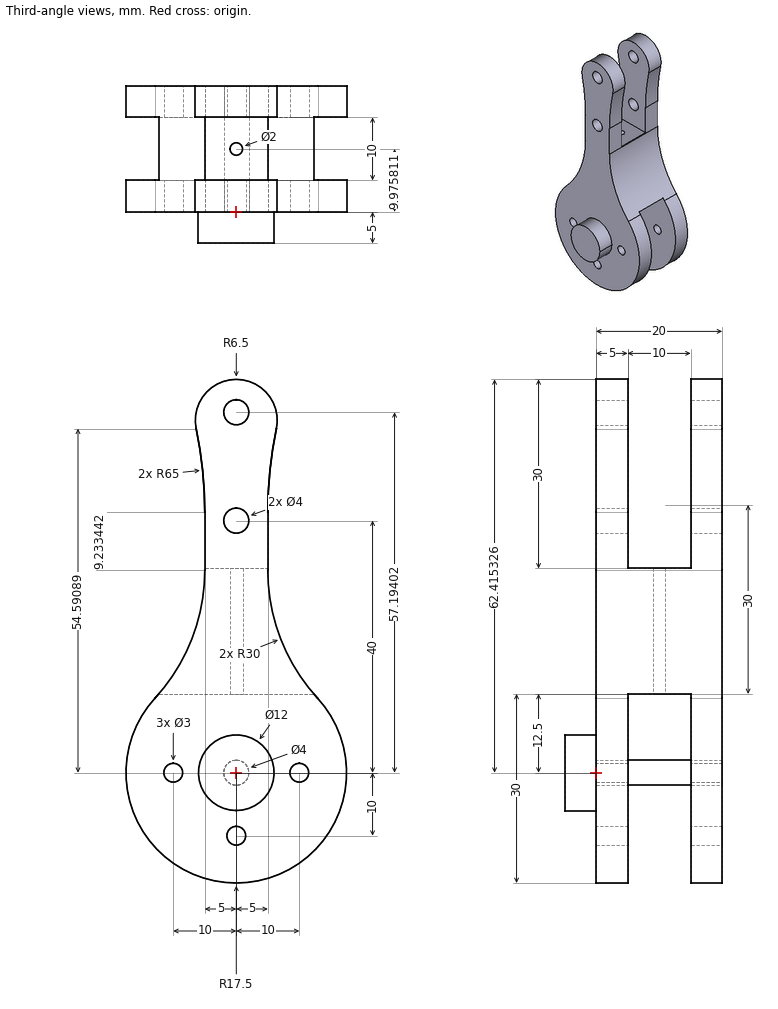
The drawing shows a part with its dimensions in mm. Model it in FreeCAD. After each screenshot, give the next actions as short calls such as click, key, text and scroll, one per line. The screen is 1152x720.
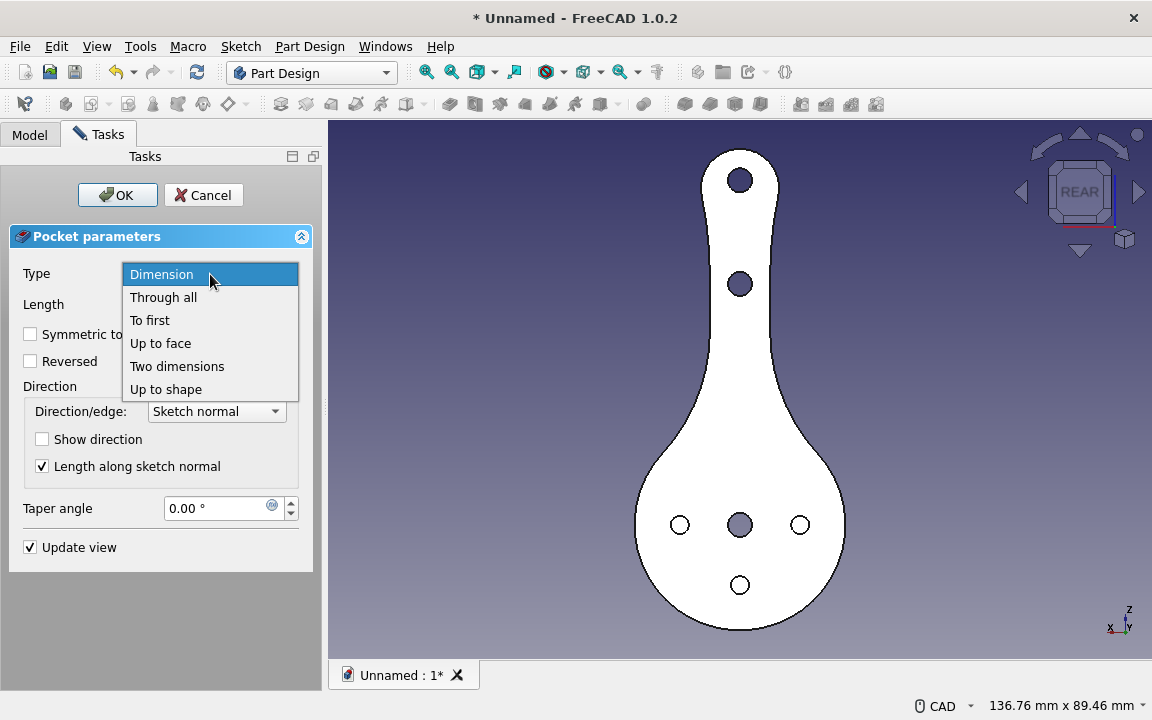
click(208, 298)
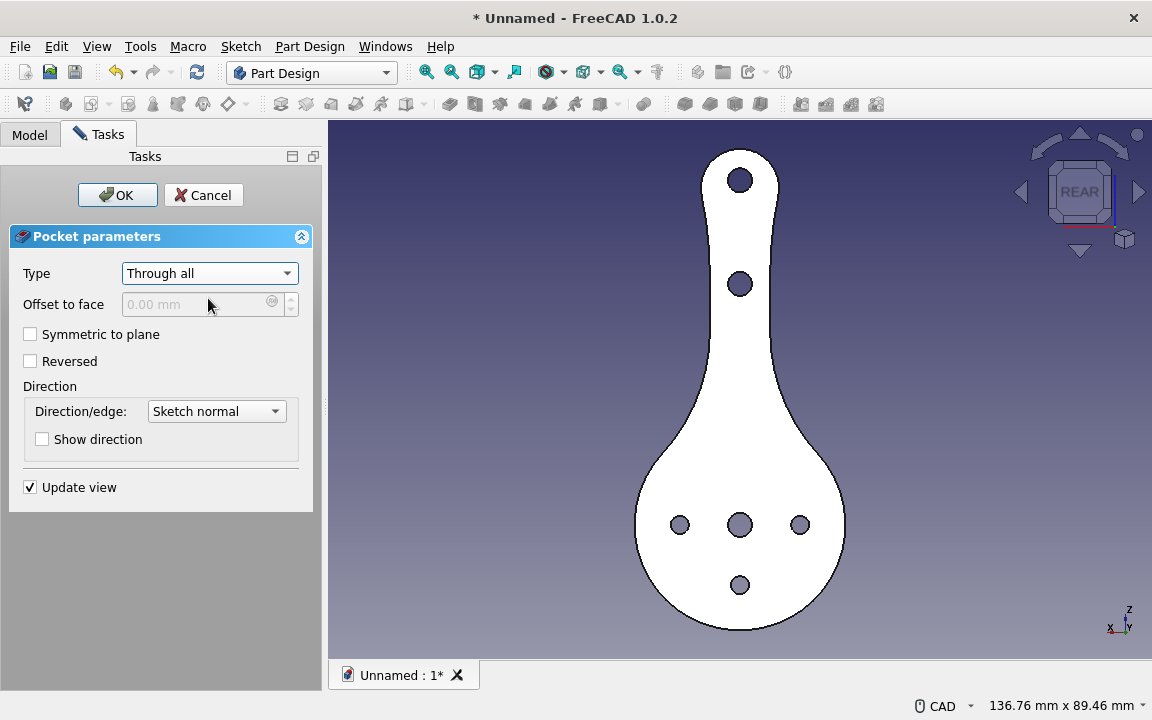
click(118, 195)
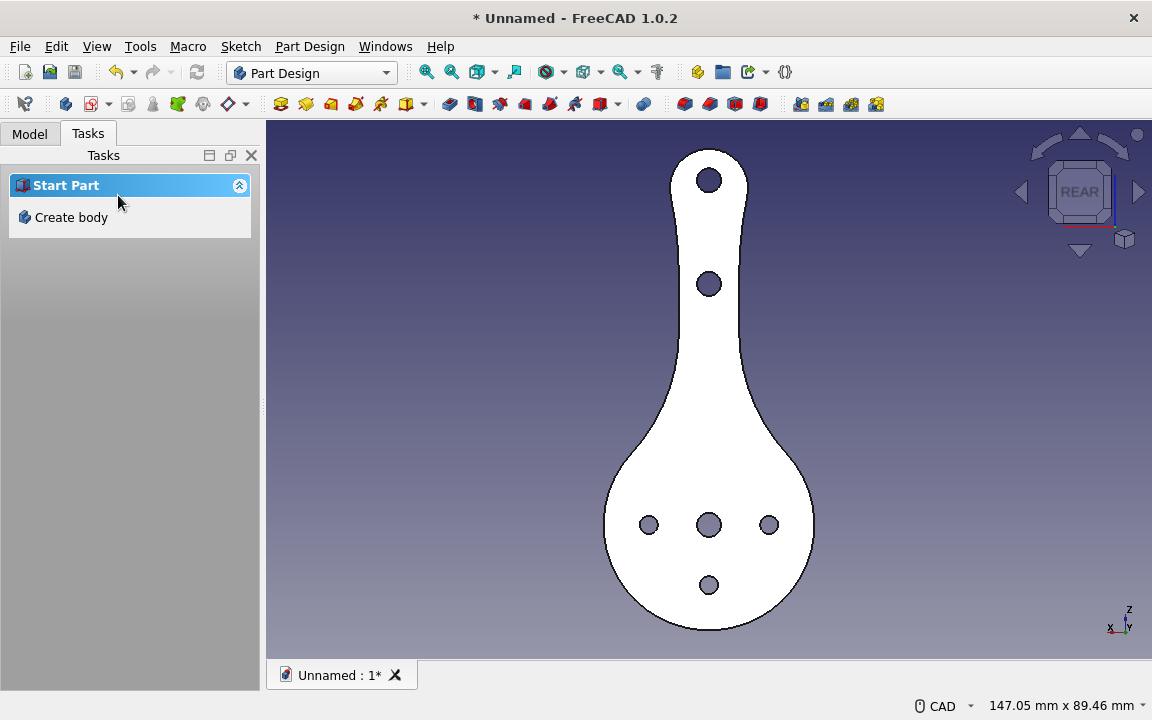
click(90, 104)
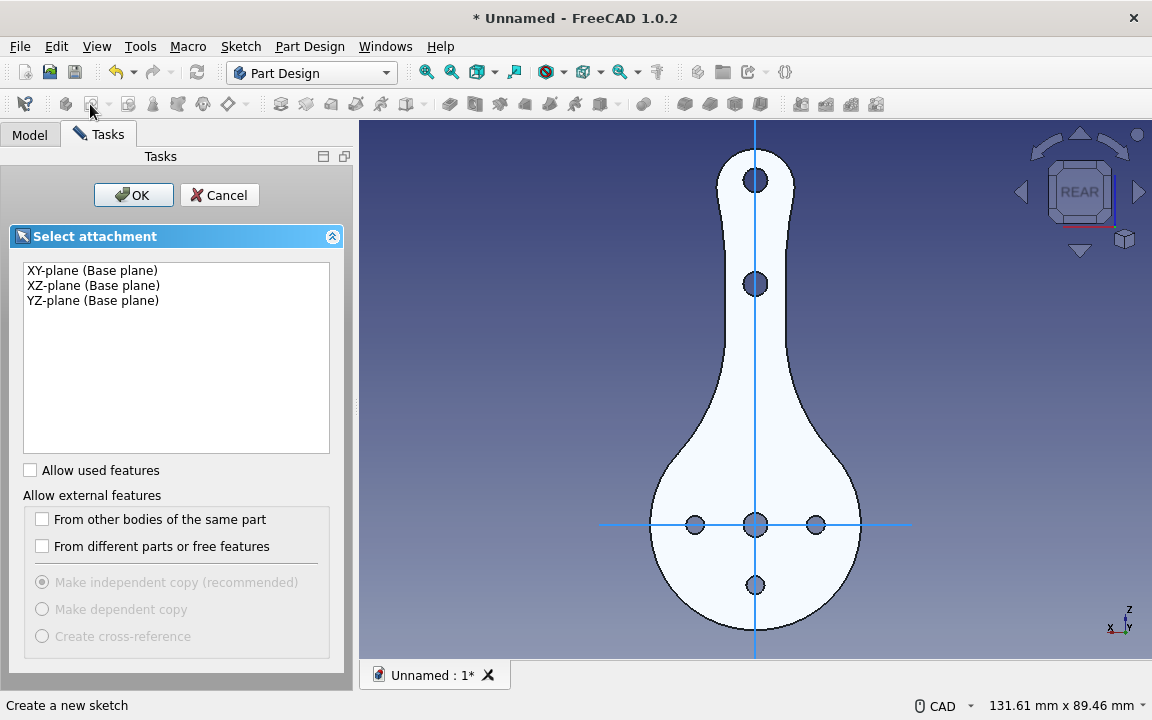
click(84, 300)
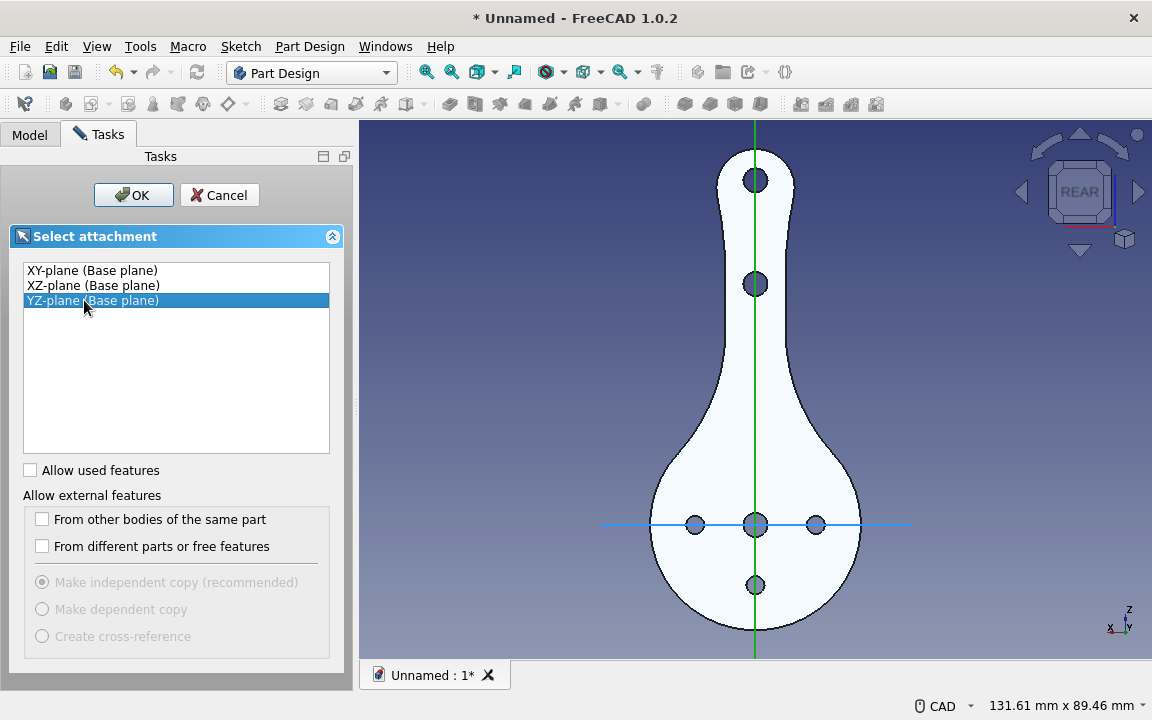
click(134, 195)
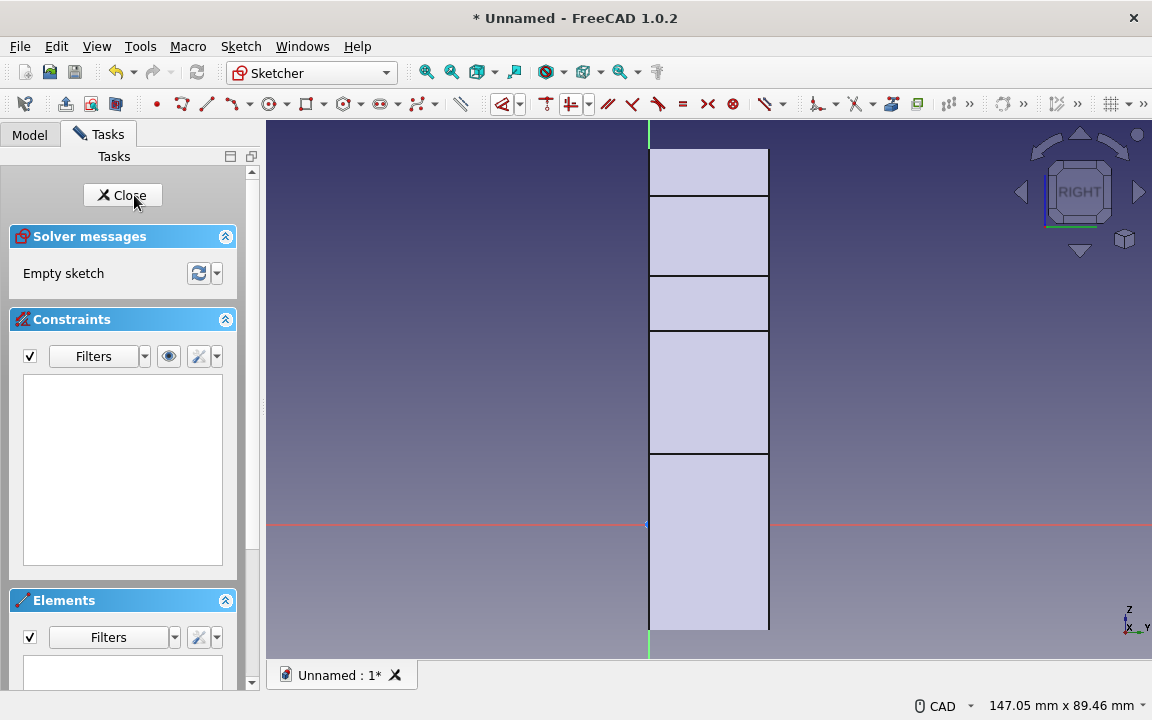
click(116, 104)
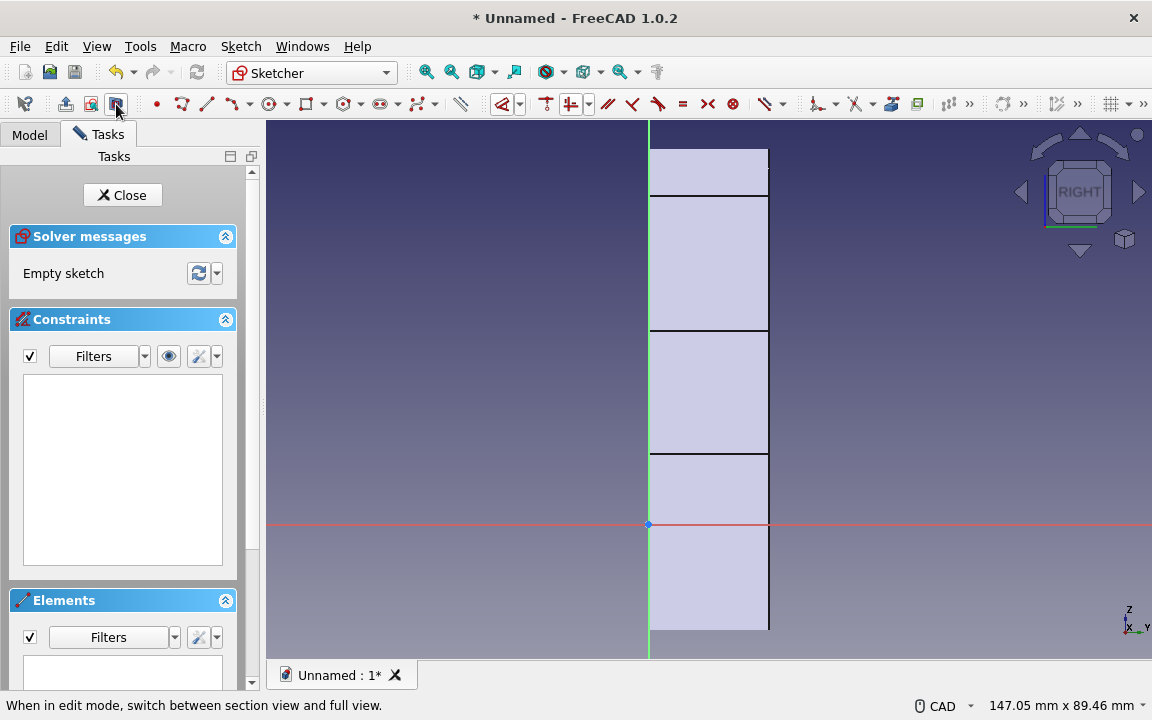
scroll(532, 389, down, 2)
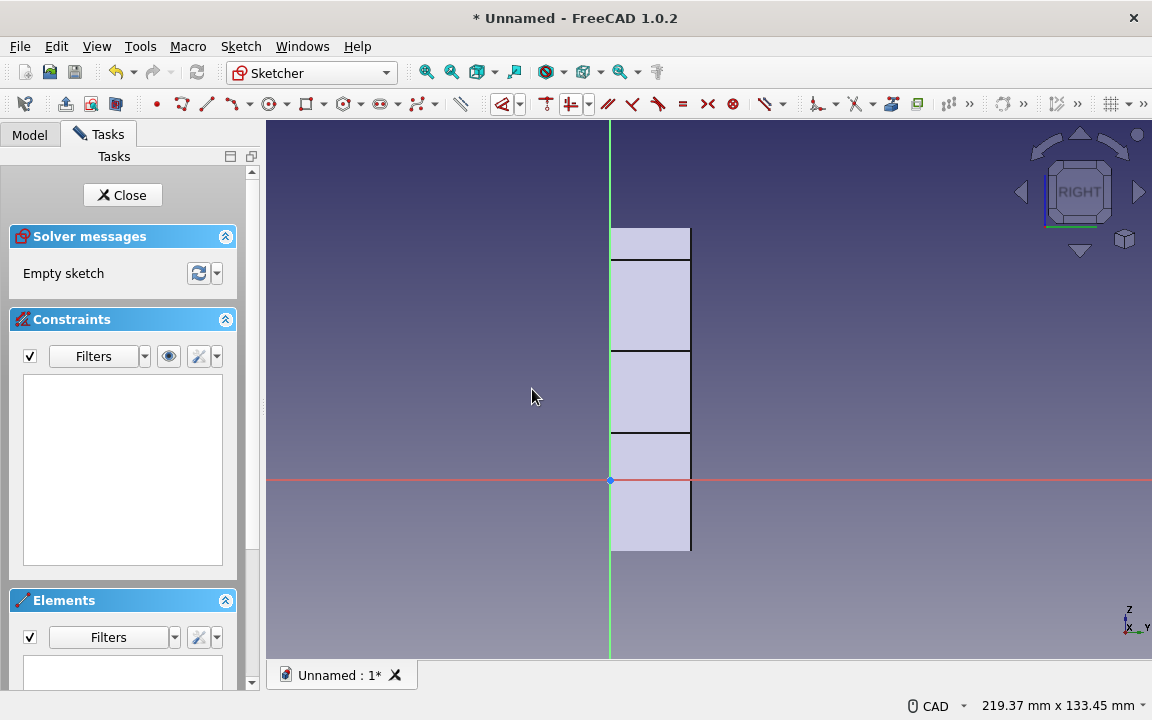
click(306, 104)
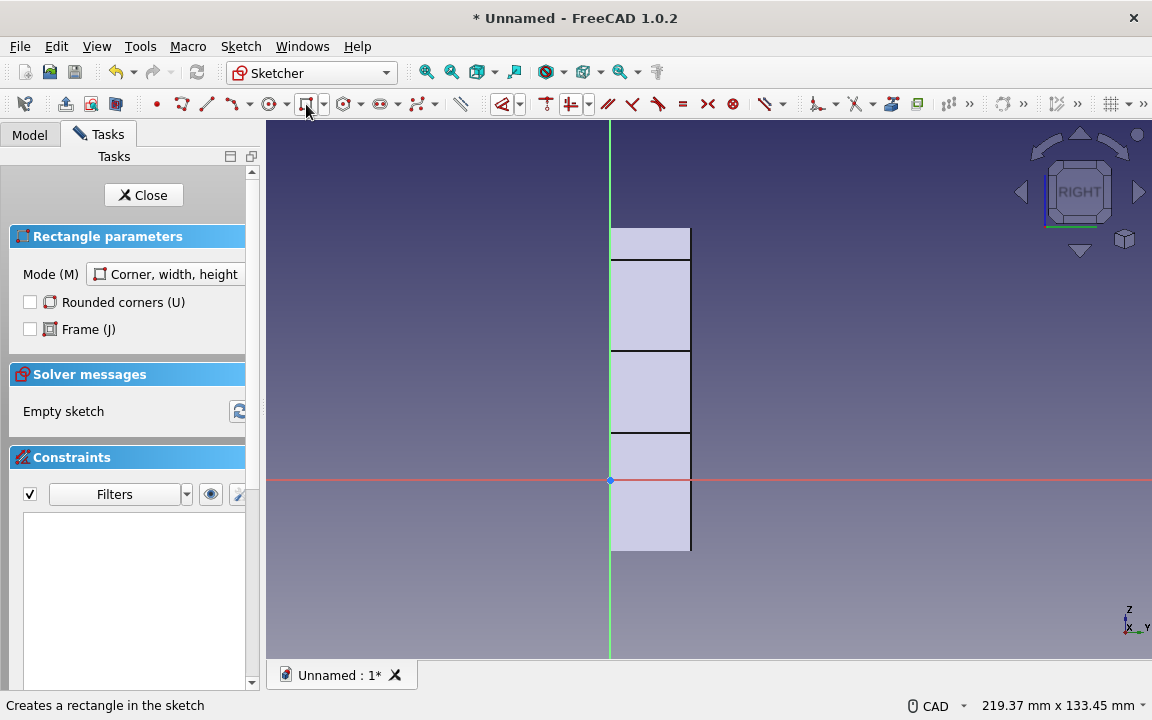
click(631, 228)
click(671, 349)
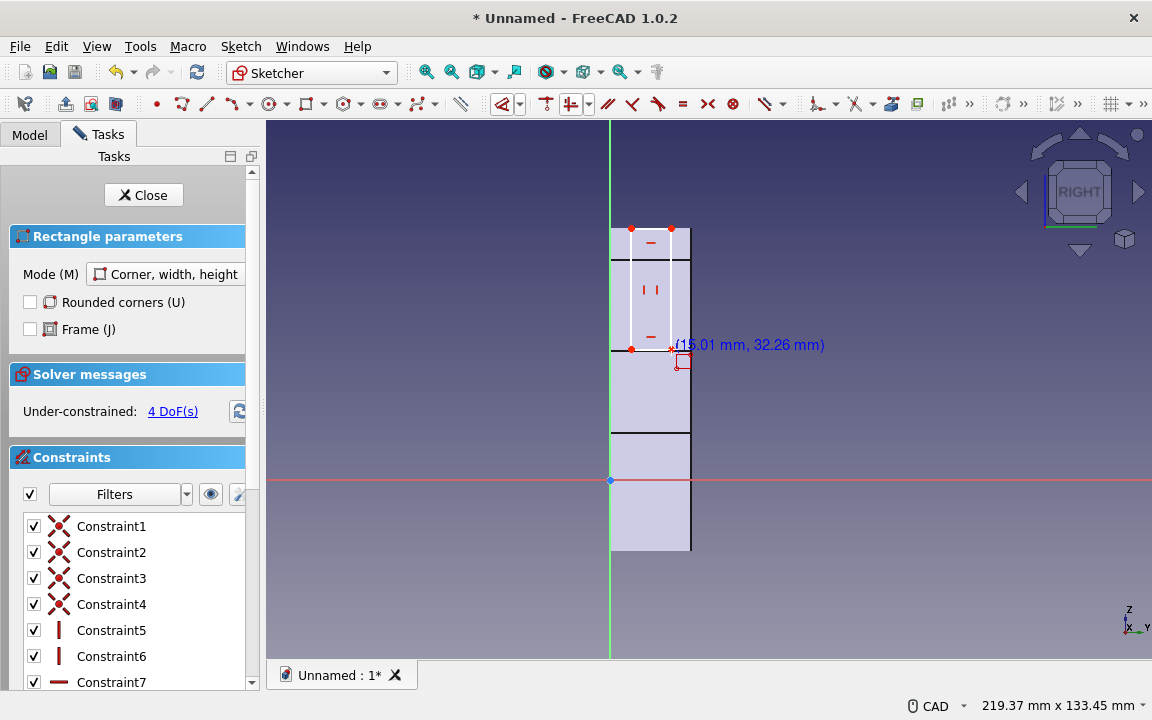
click(631, 430)
click(671, 551)
key(Escape)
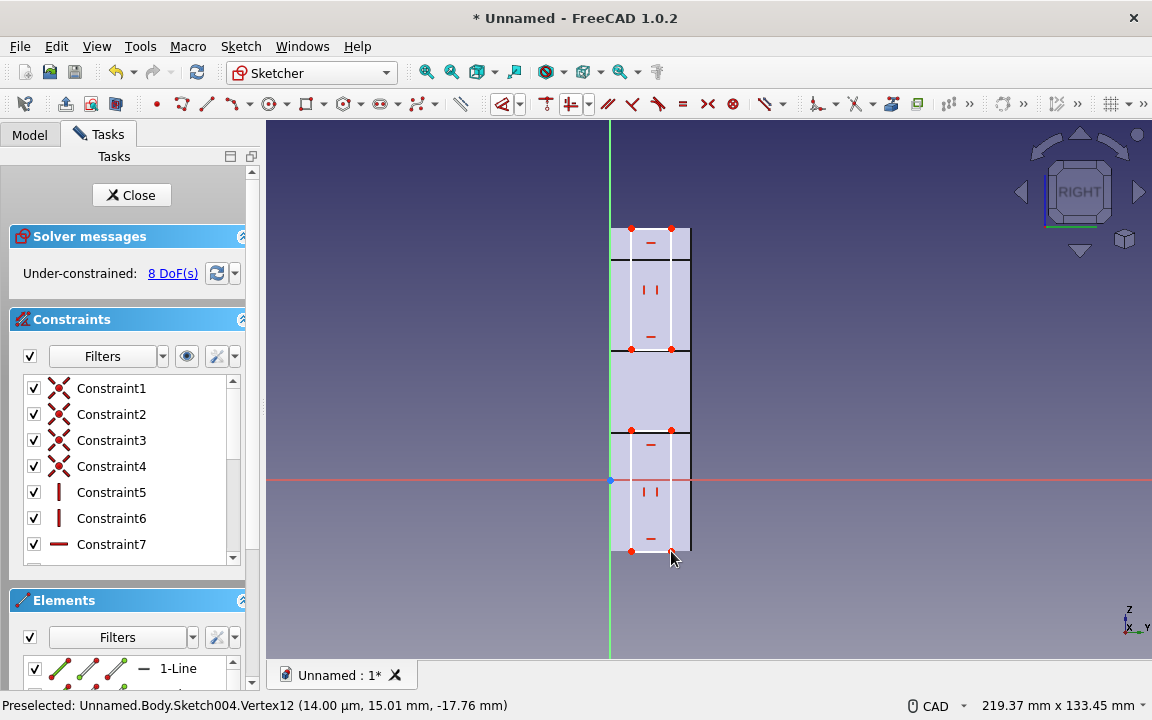
click(631, 265)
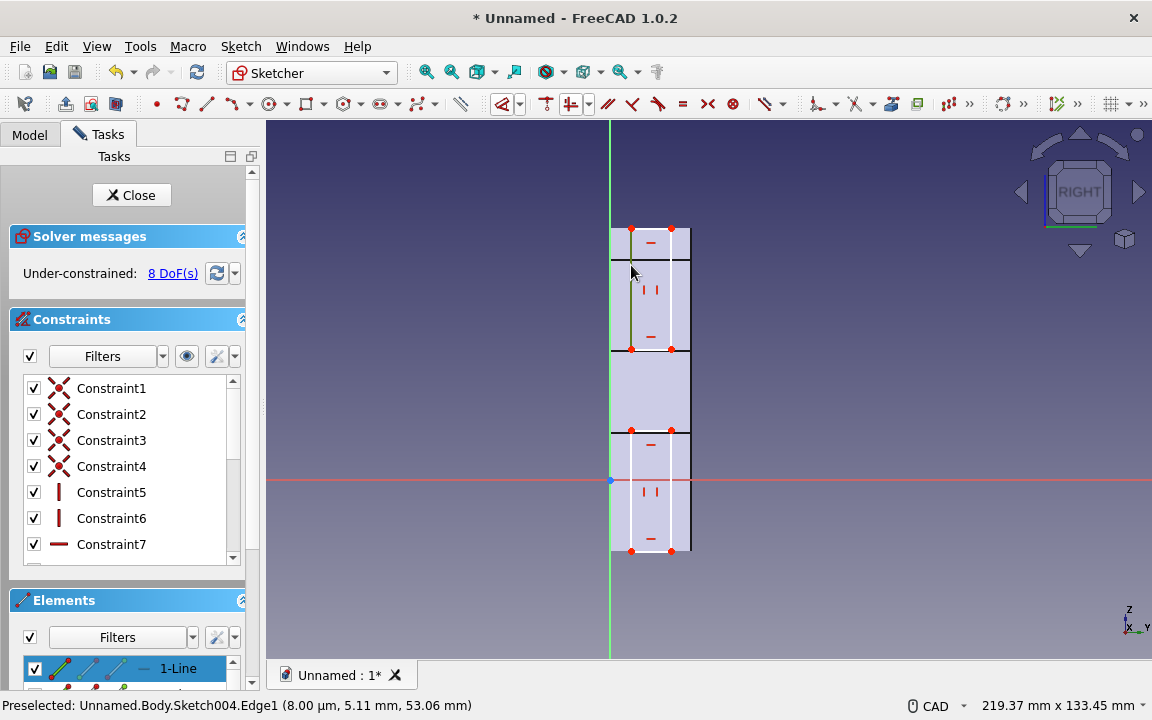
click(520, 104)